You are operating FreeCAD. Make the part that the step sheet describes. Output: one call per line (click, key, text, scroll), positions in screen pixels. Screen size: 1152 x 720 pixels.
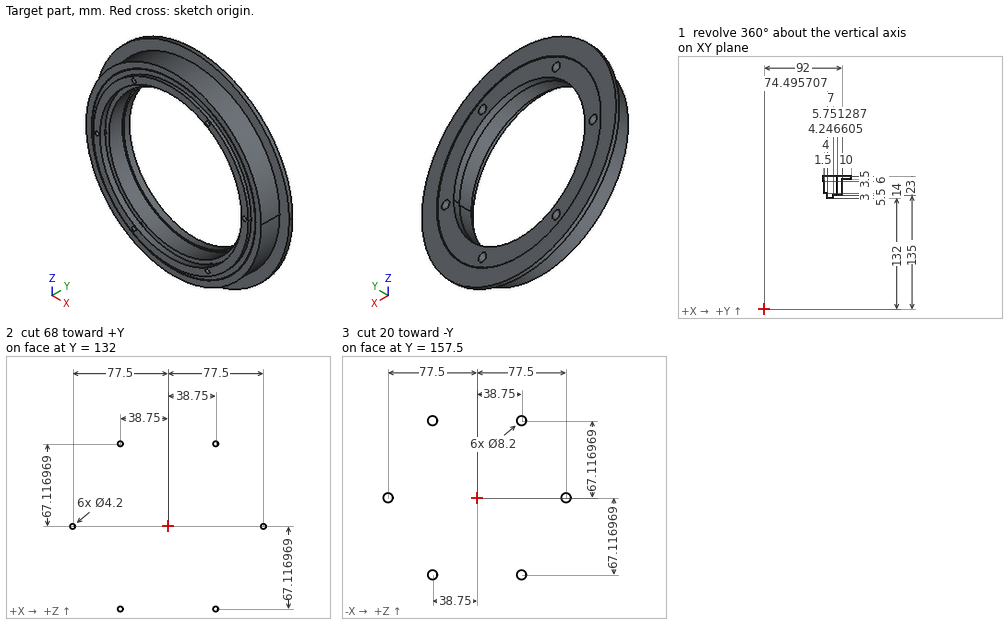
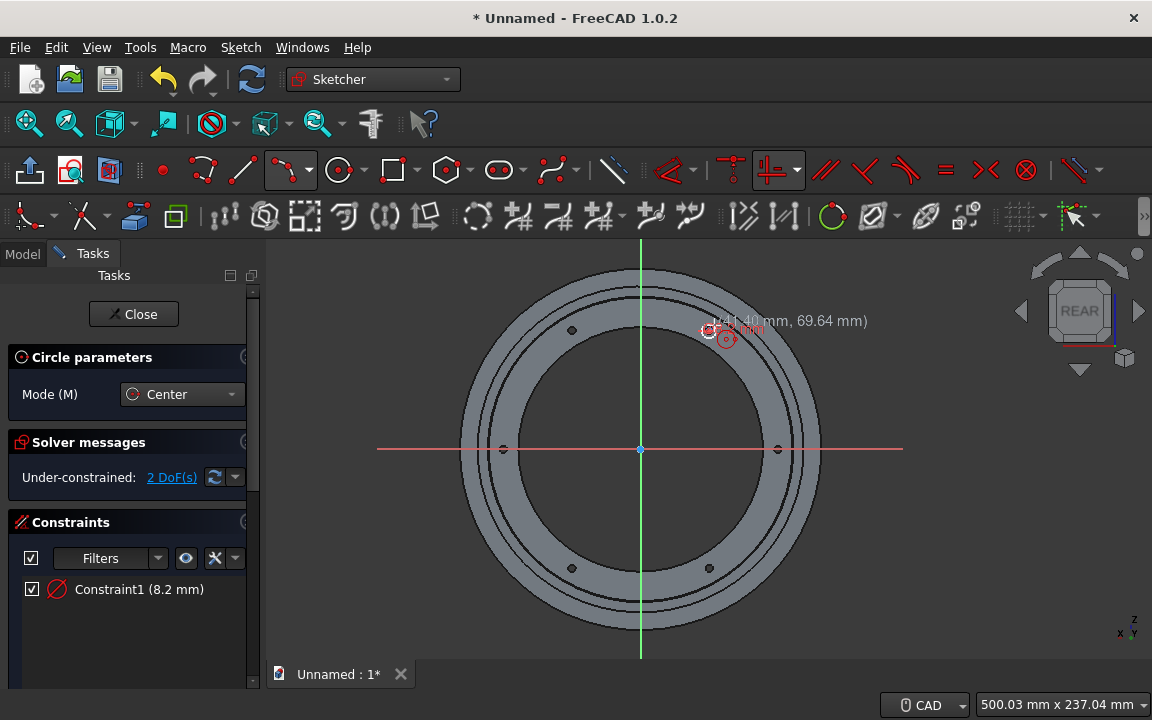
scroll(778, 449, up, 6)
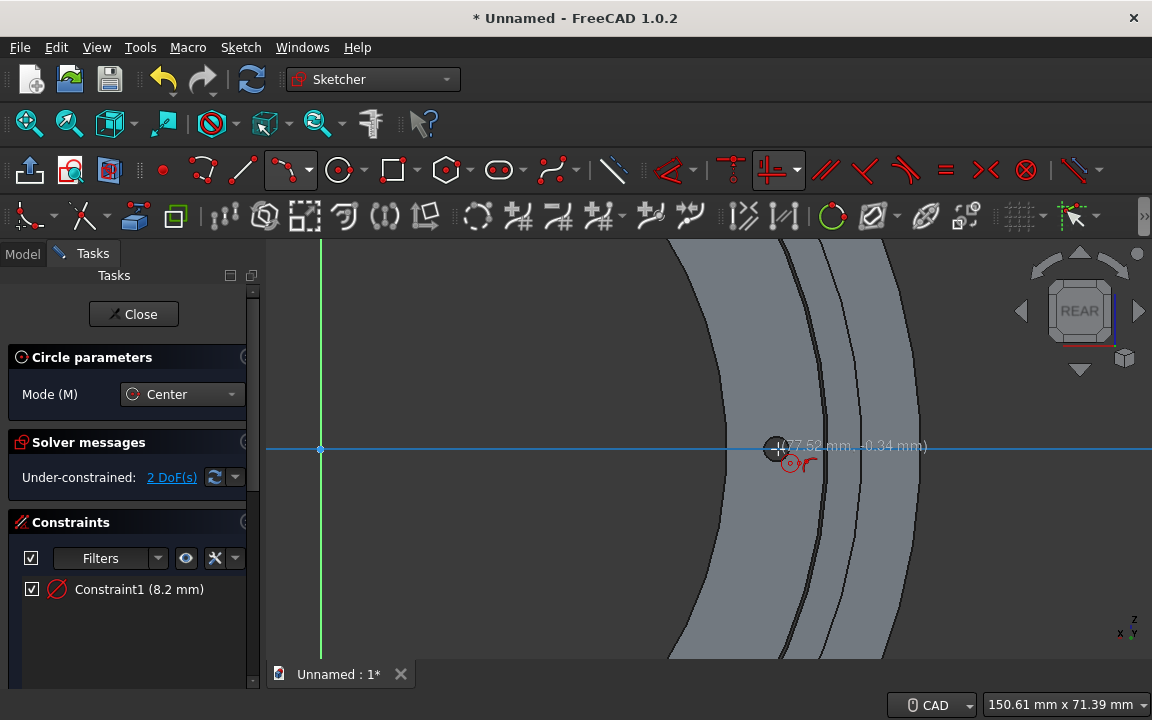
scroll(778, 449, down, 6)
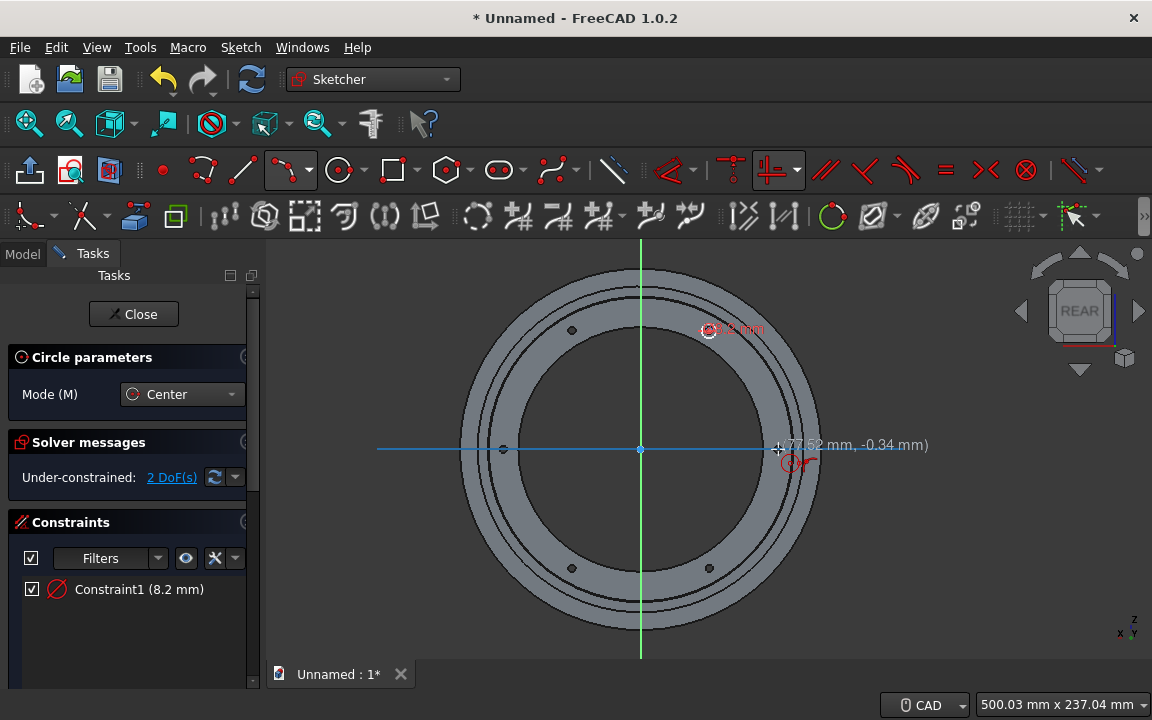
click(778, 449)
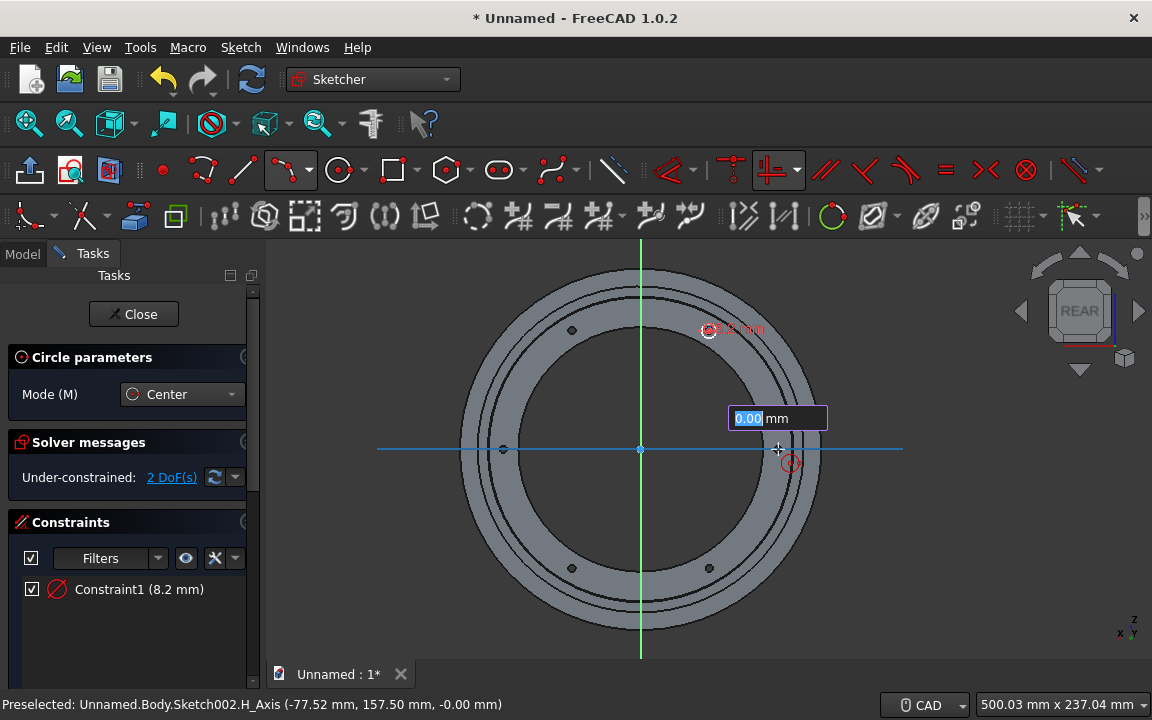
scroll(775, 456, up, 5)
move(775, 456)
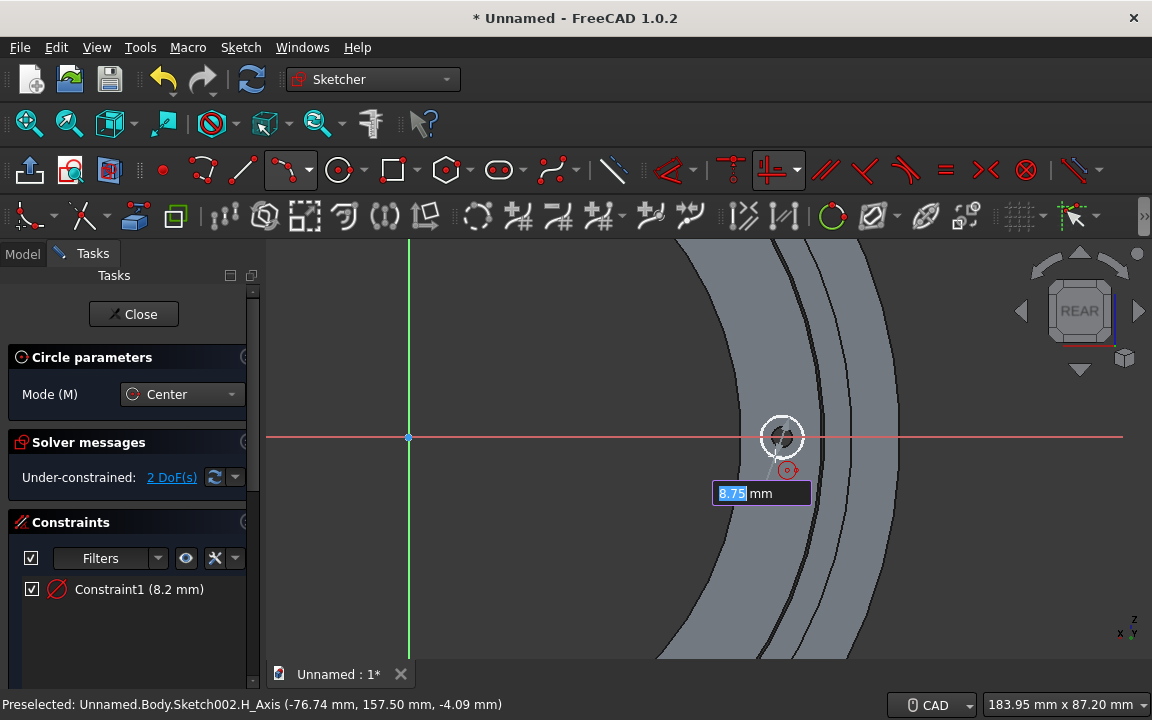
text(8.2)
key(Return)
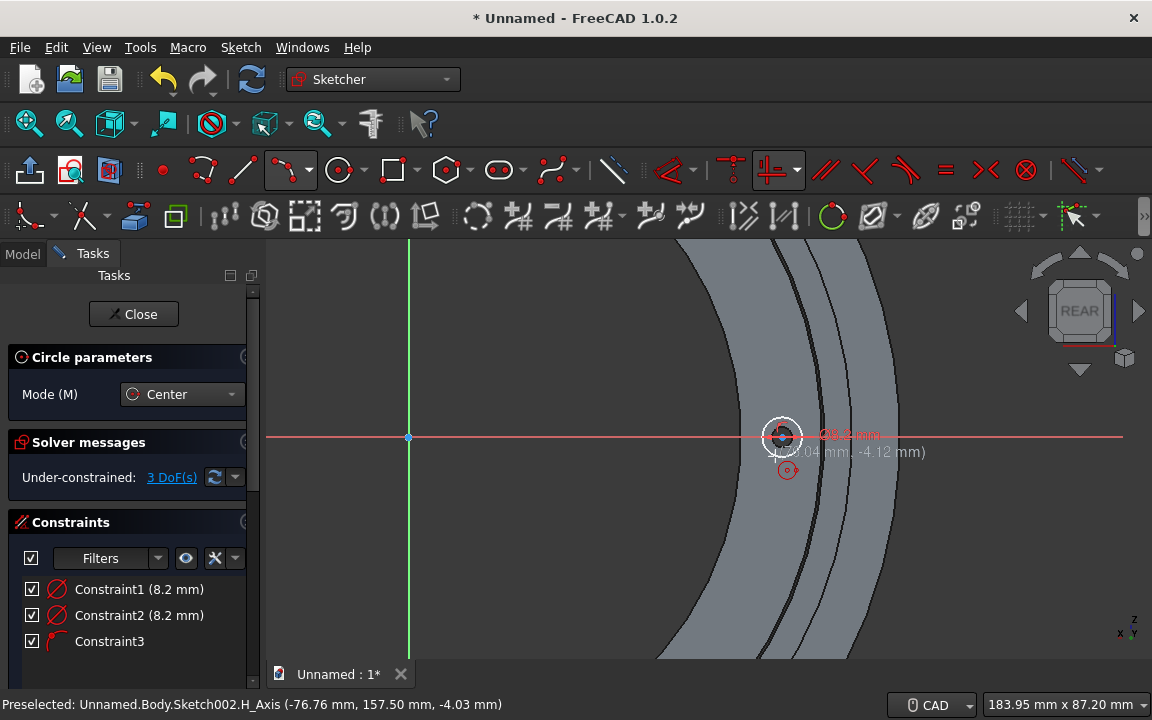
scroll(775, 456, down, 5)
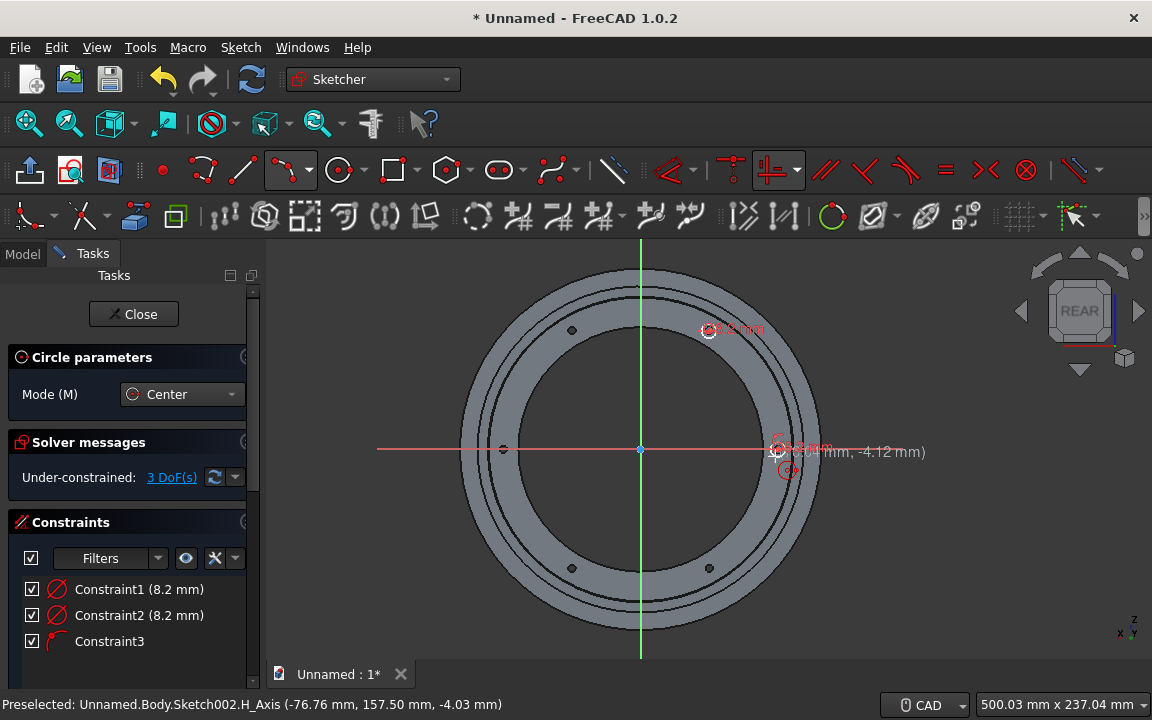
scroll(709, 568, up, 6)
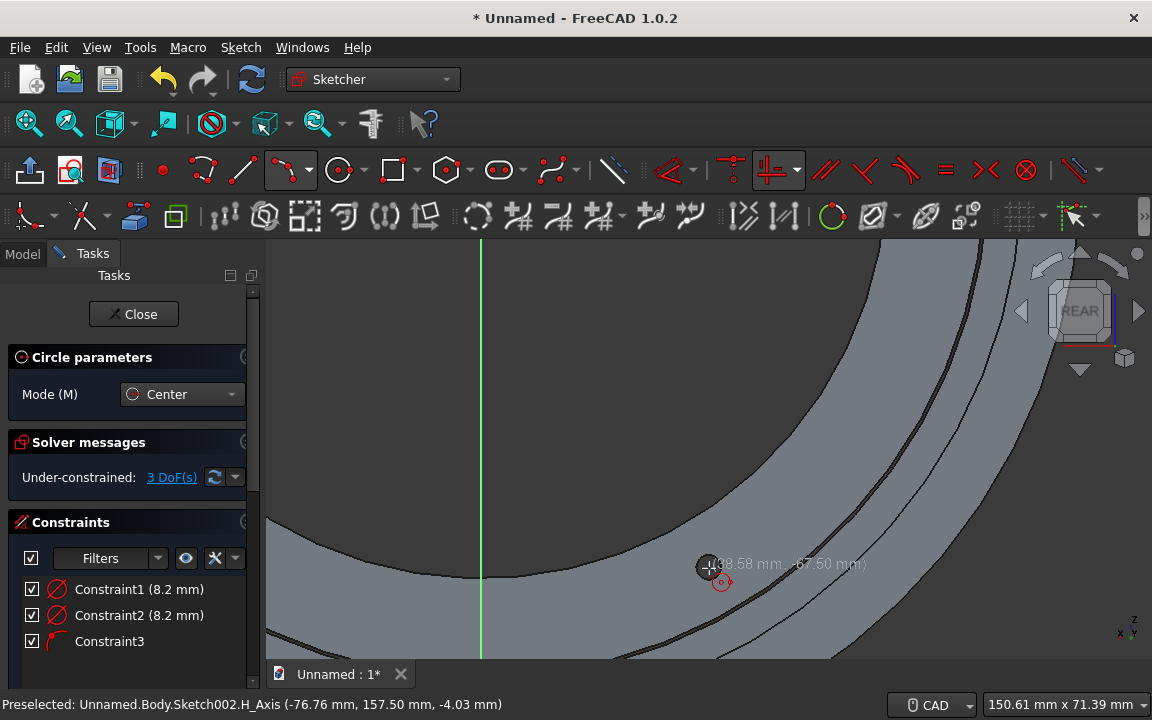
scroll(709, 568, down, 6)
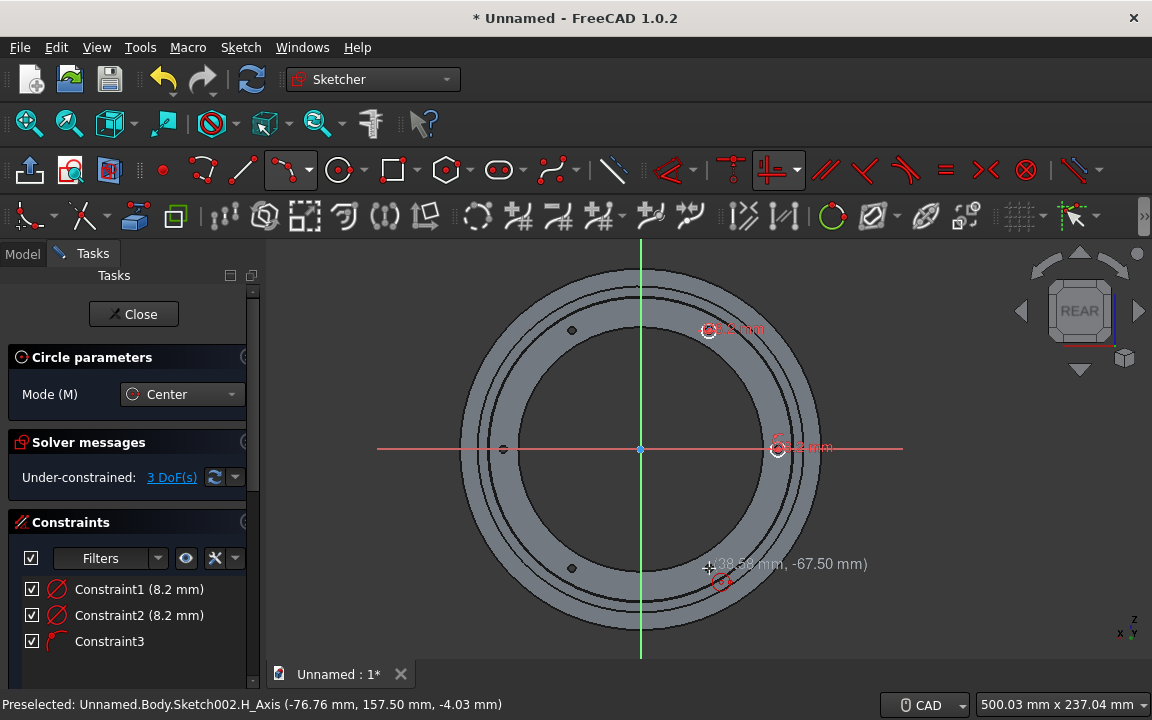
click(709, 568)
move(714, 563)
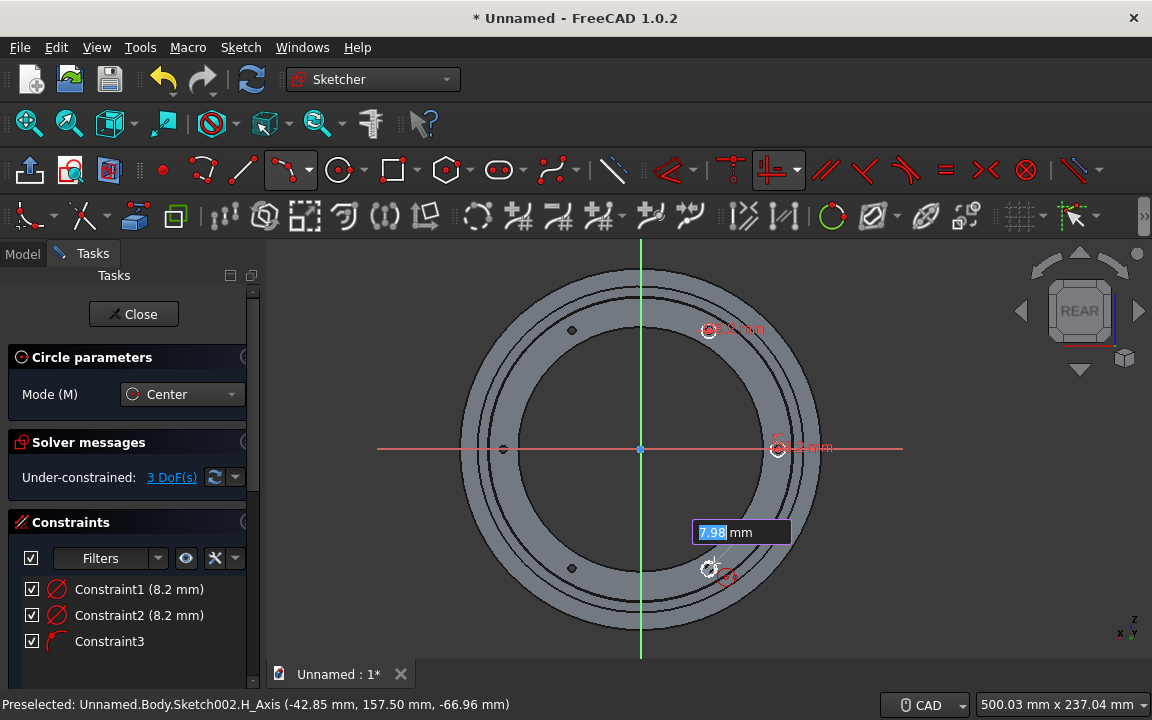
text(8.2)
key(Return)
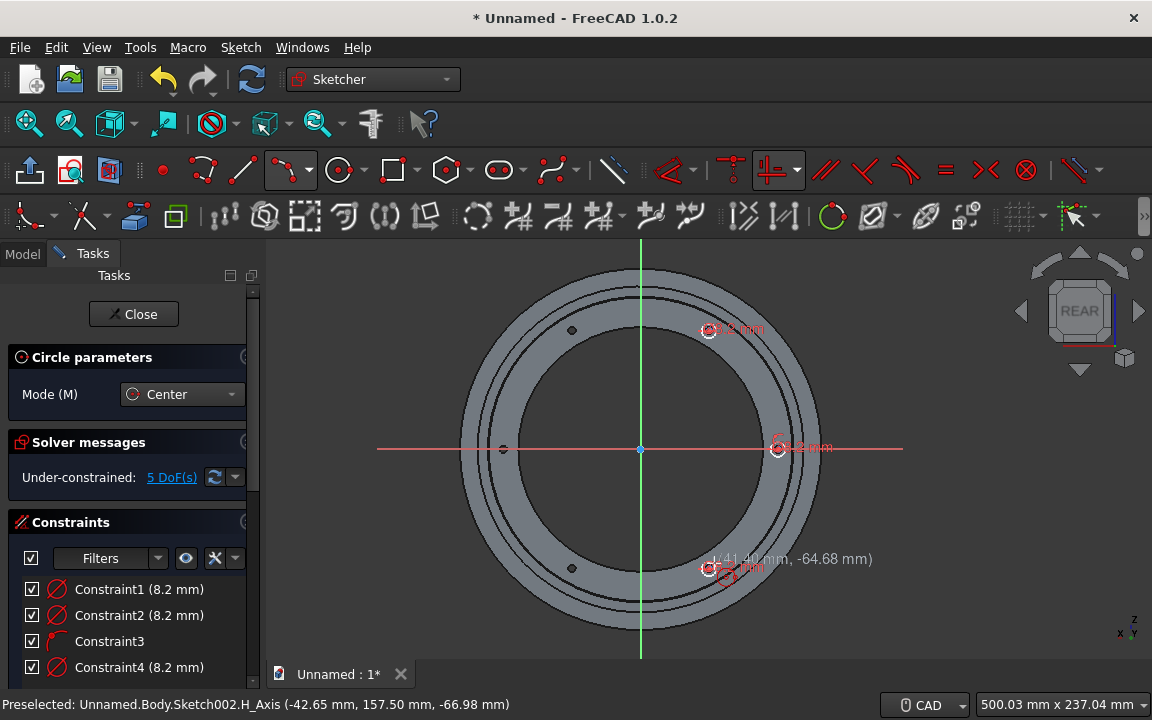
scroll(572, 568, up, 6)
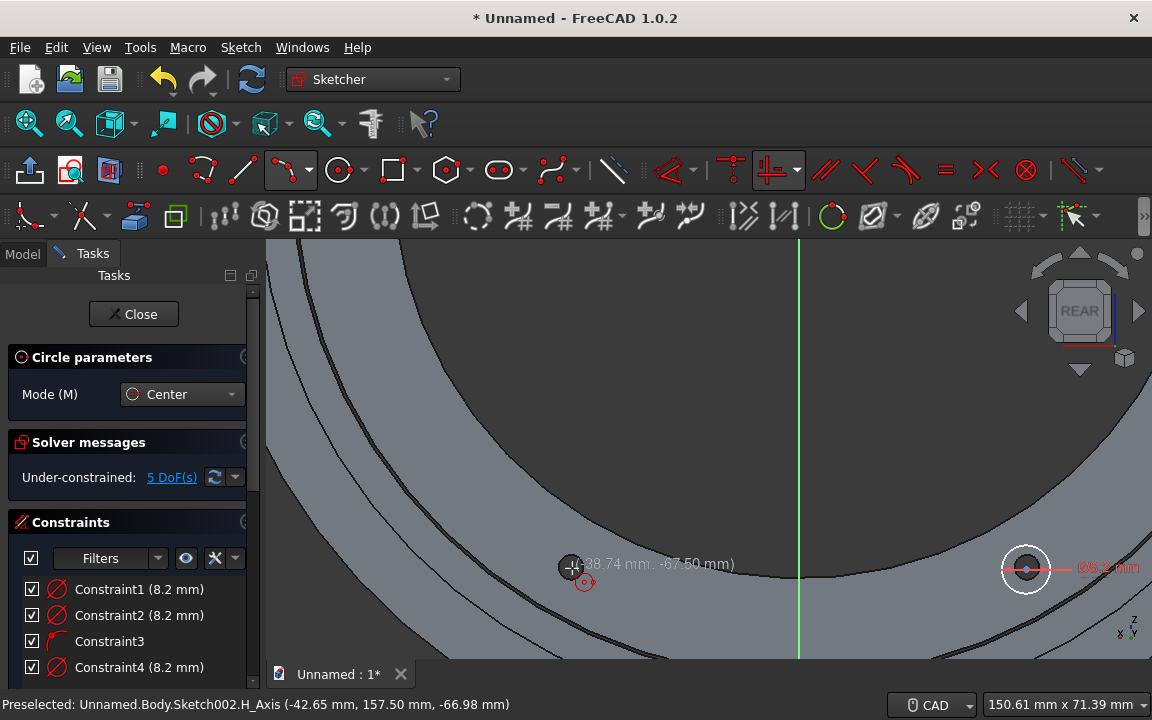
scroll(572, 568, down, 6)